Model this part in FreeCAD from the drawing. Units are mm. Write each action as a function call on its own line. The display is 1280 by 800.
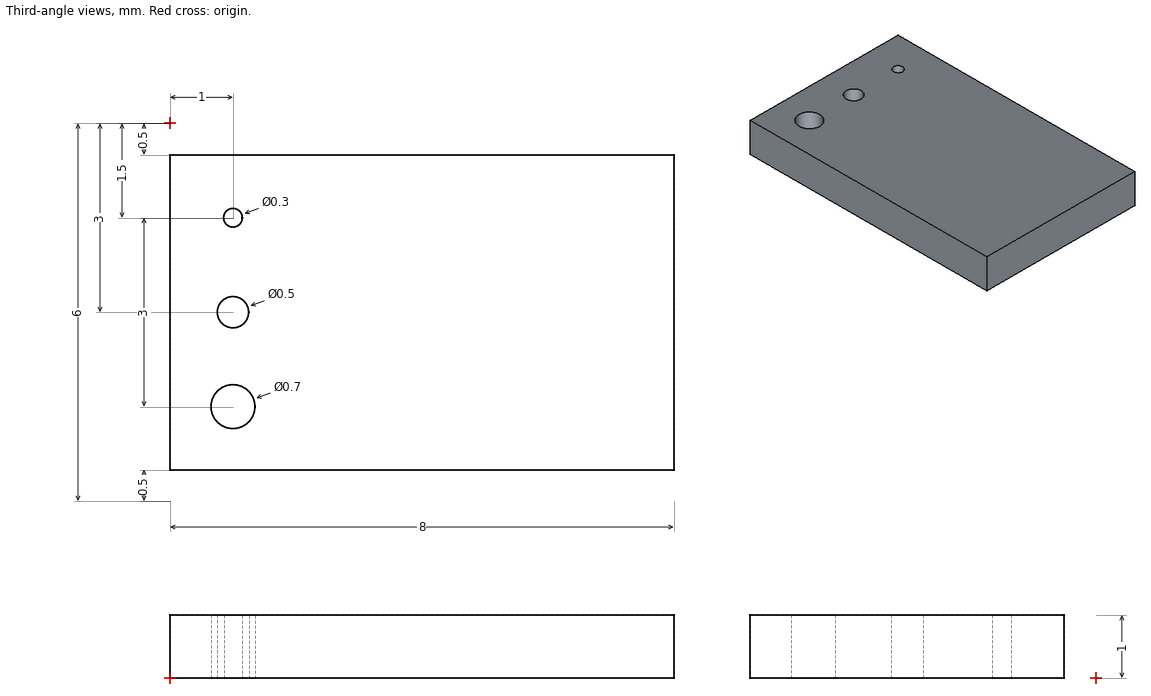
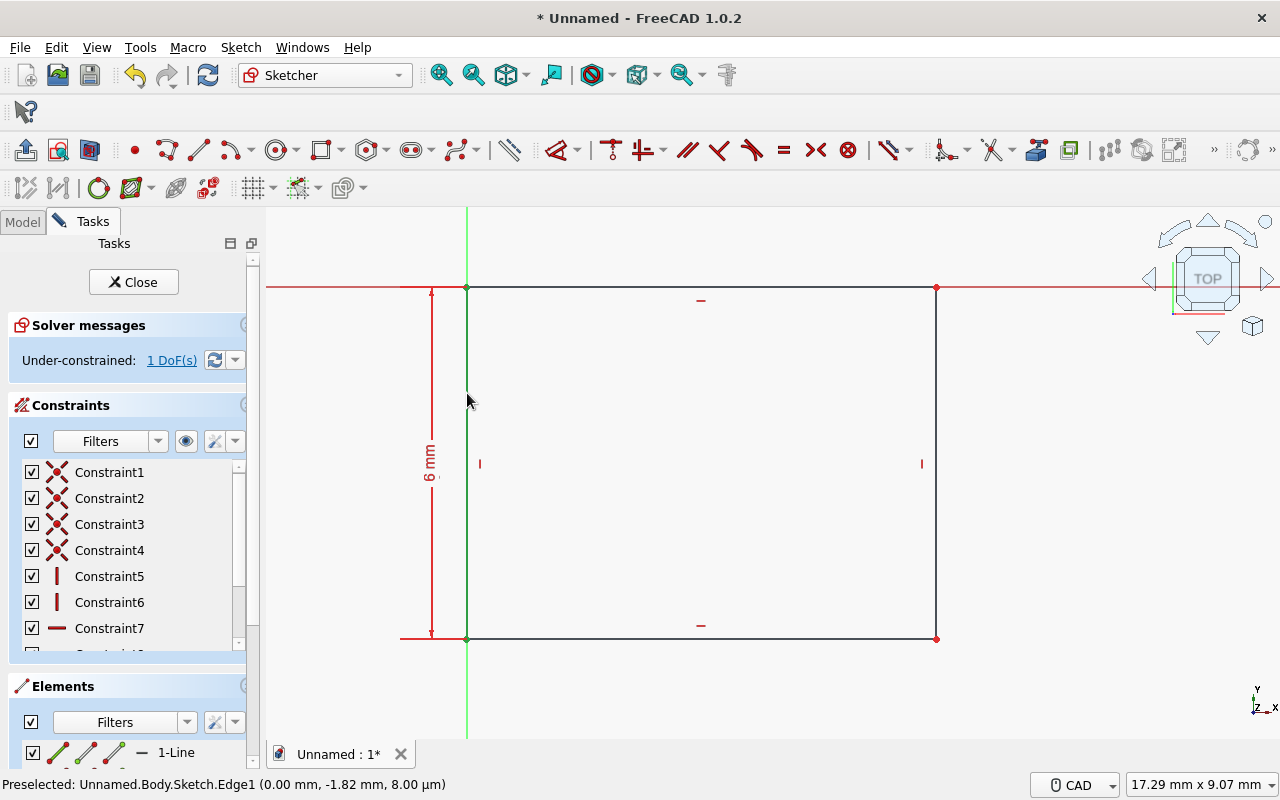
click(608, 639)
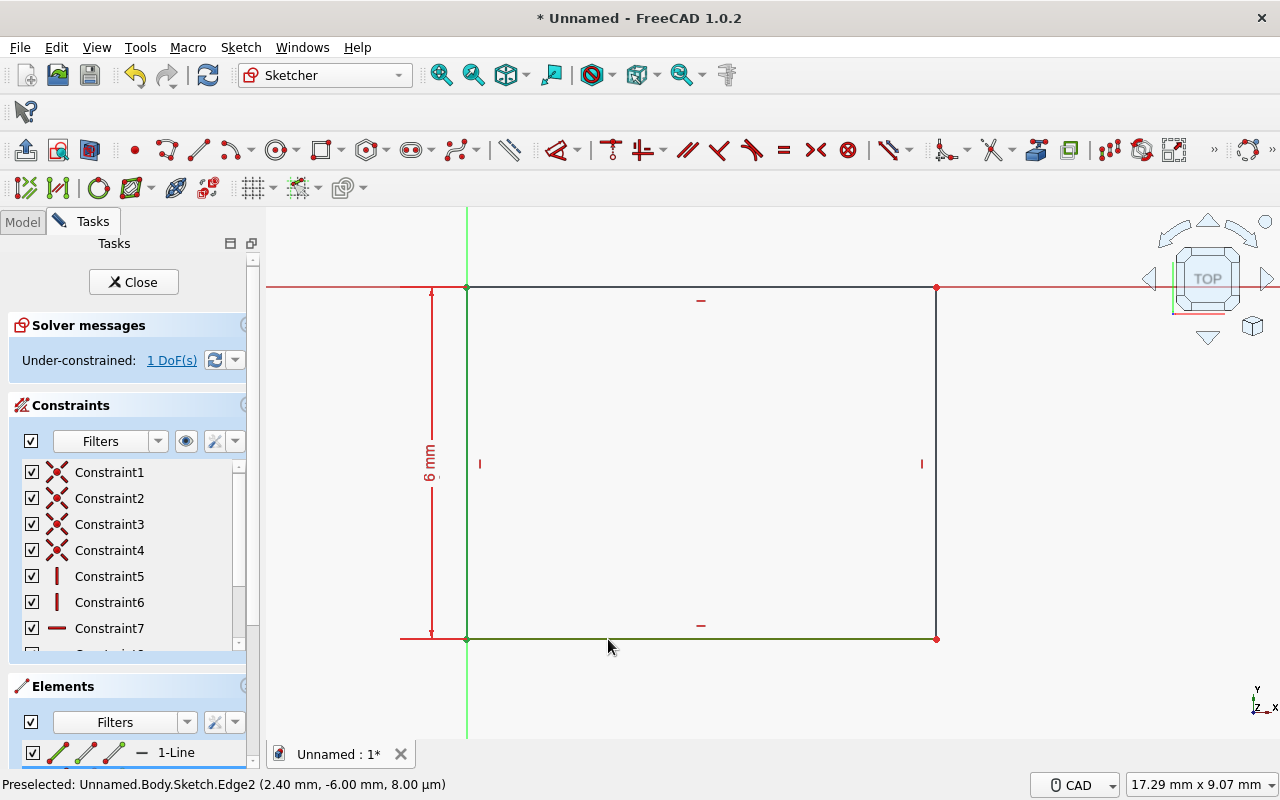
click(580, 150)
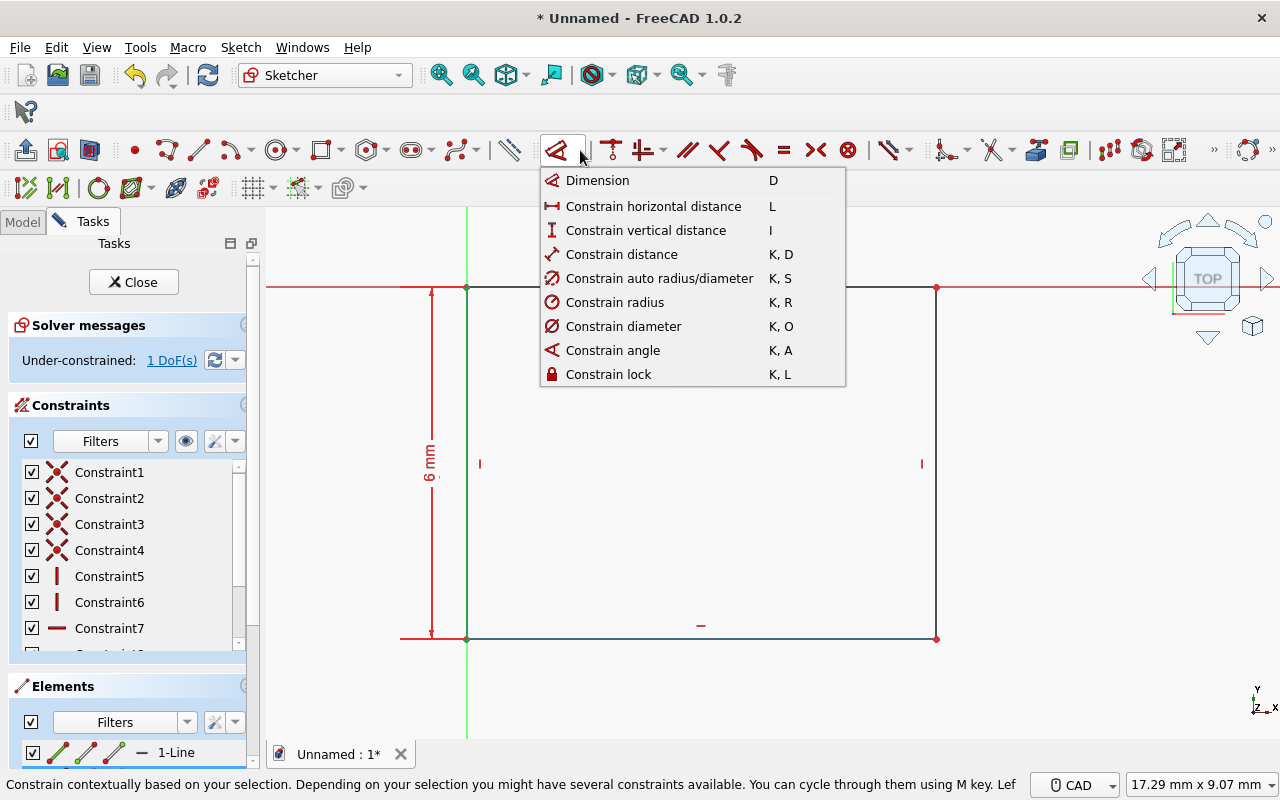
click(693, 206)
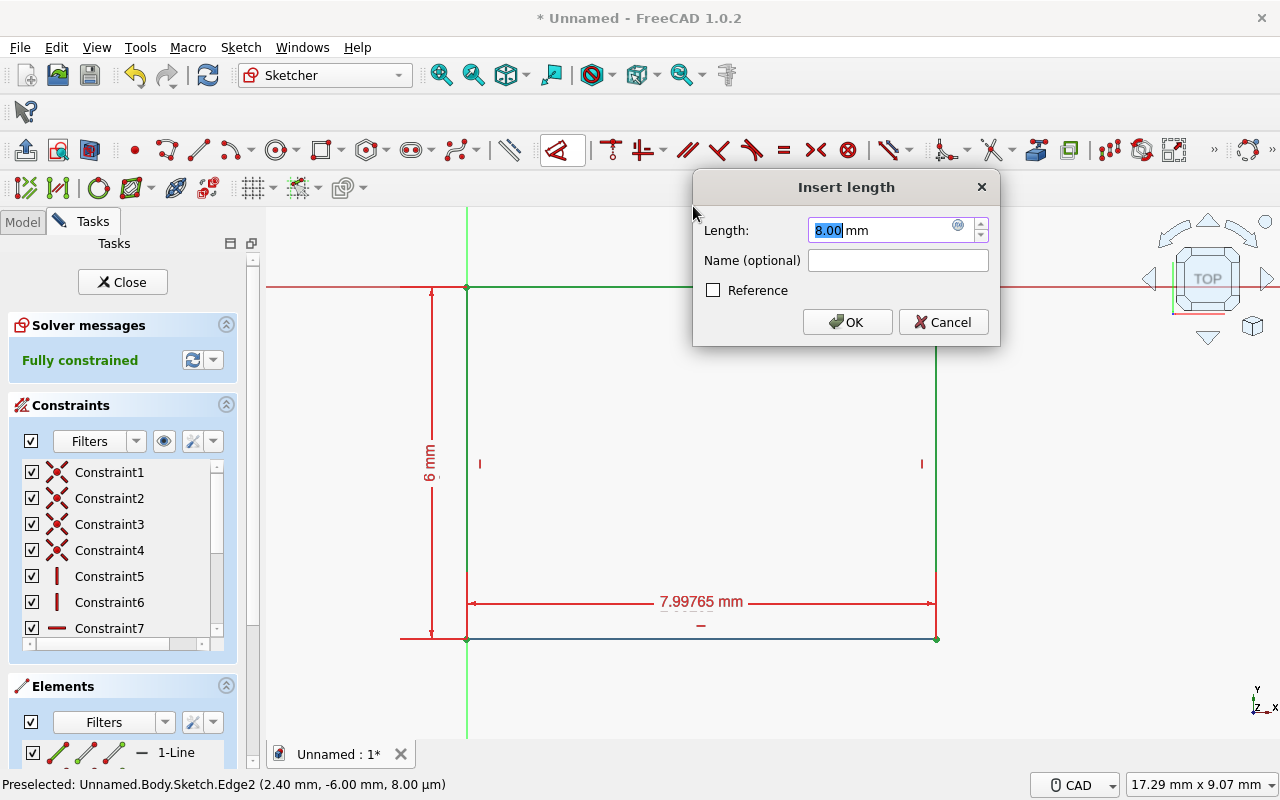
text(8)
key(Return)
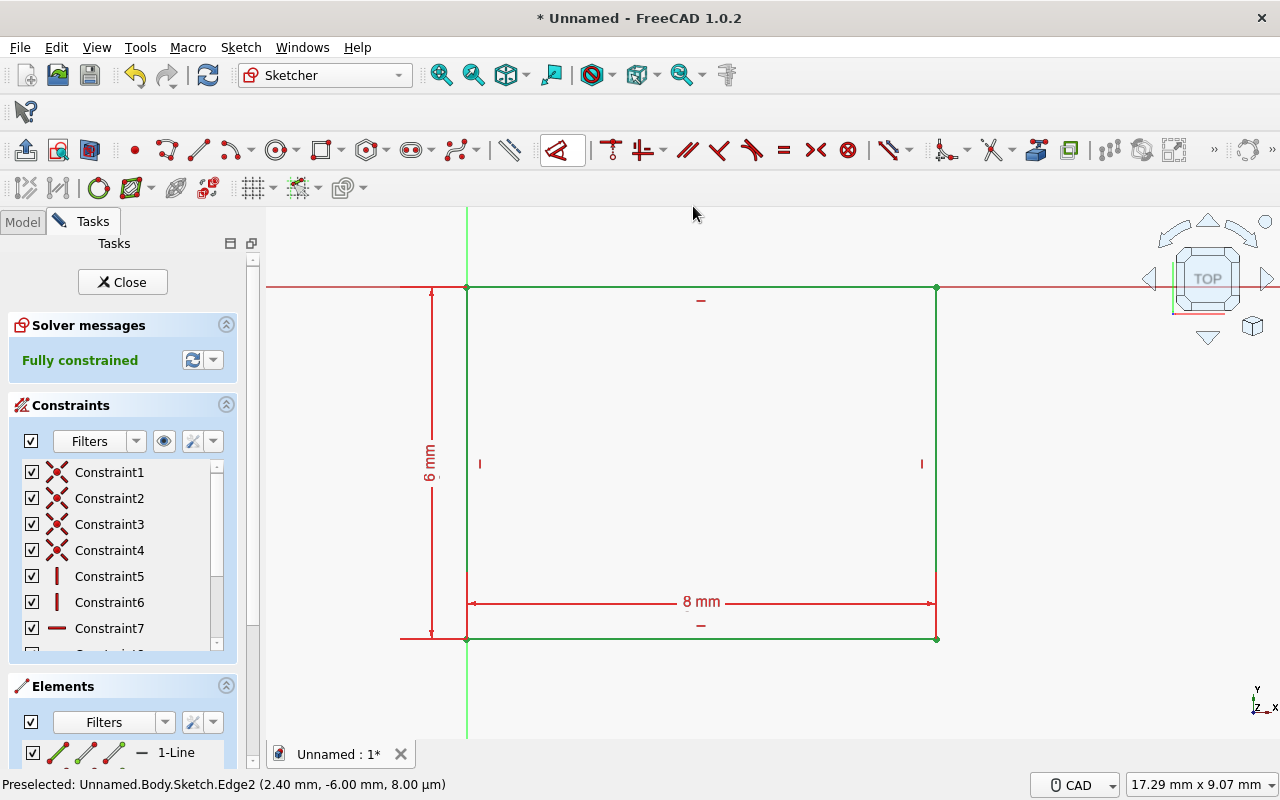
click(123, 282)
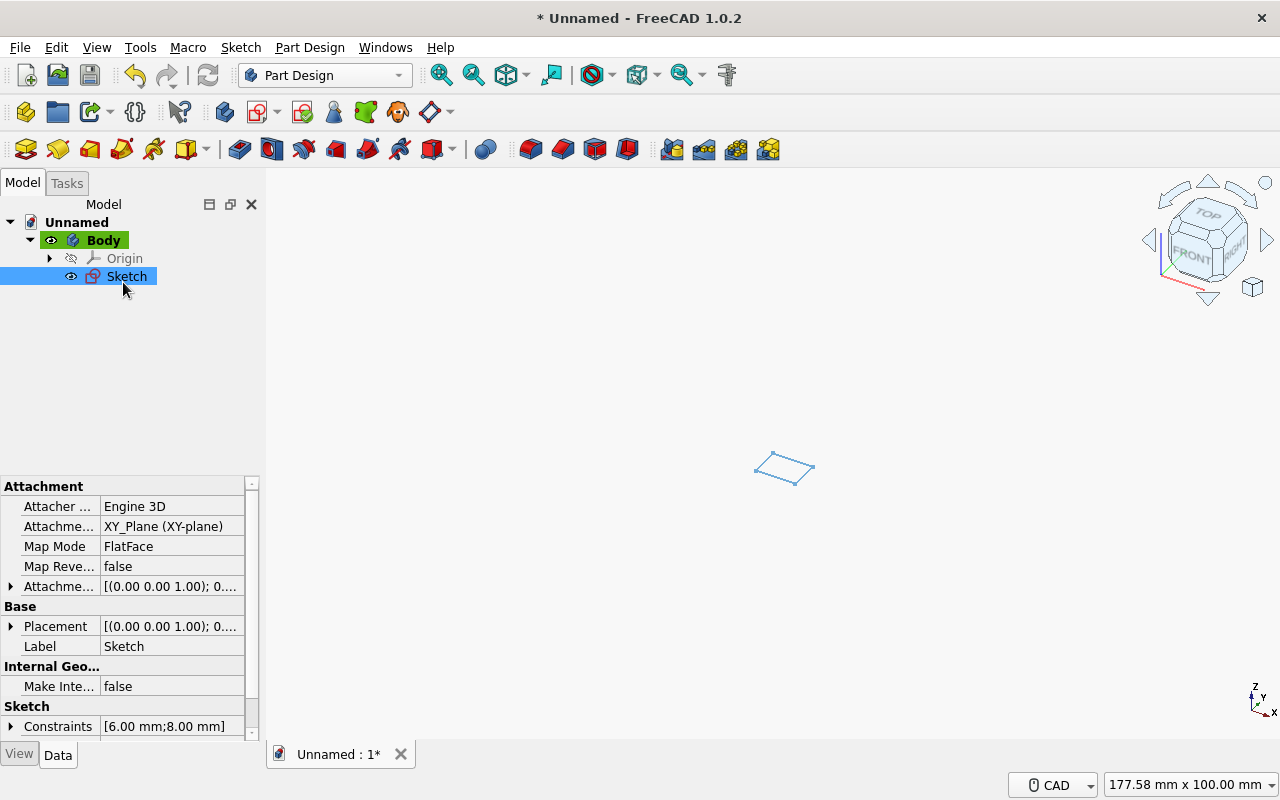
click(26, 150)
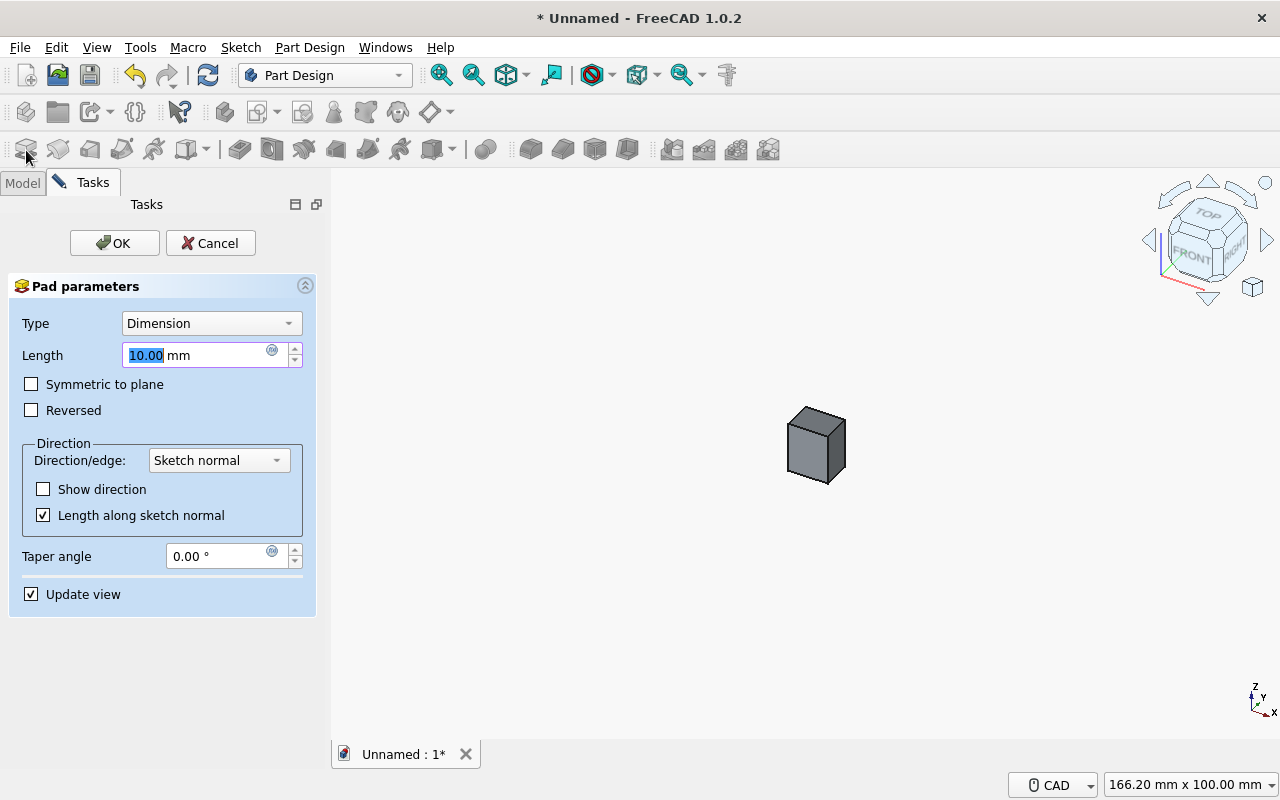
text(1)
key(Tab)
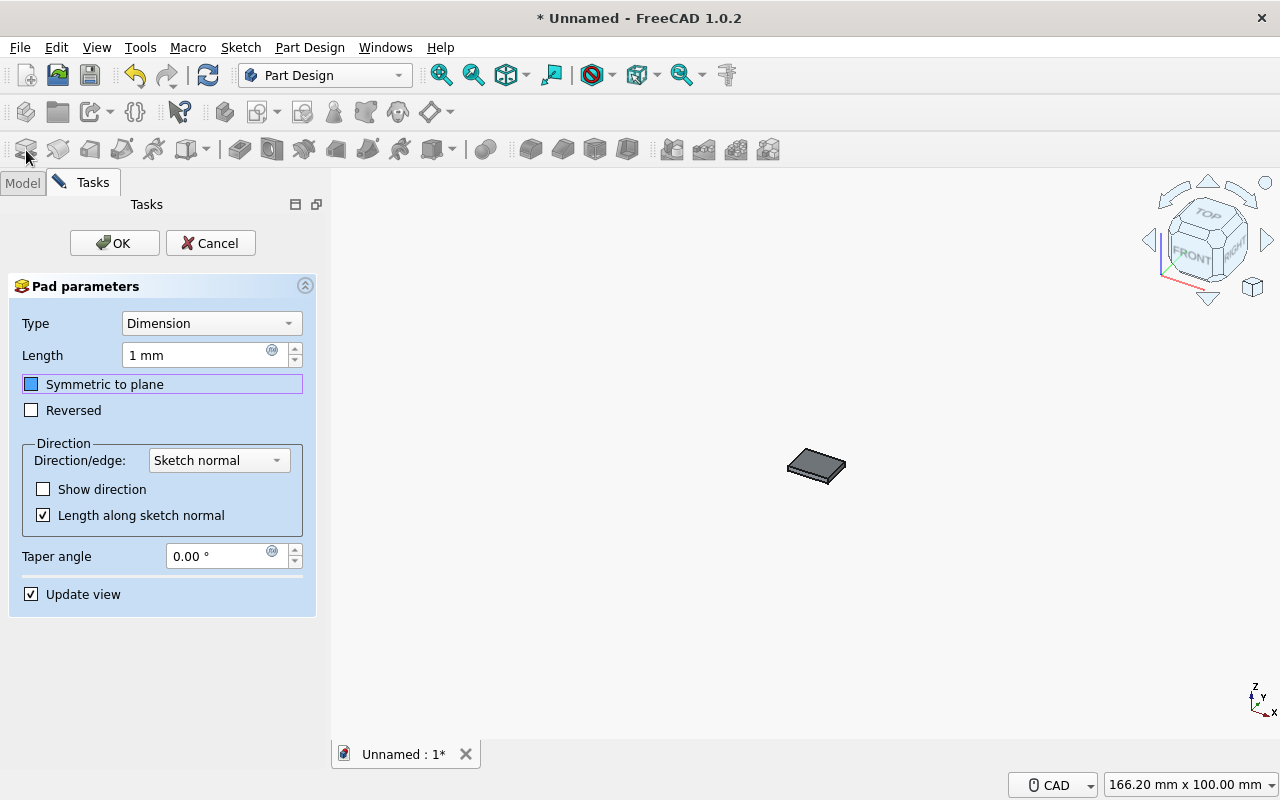
click(115, 243)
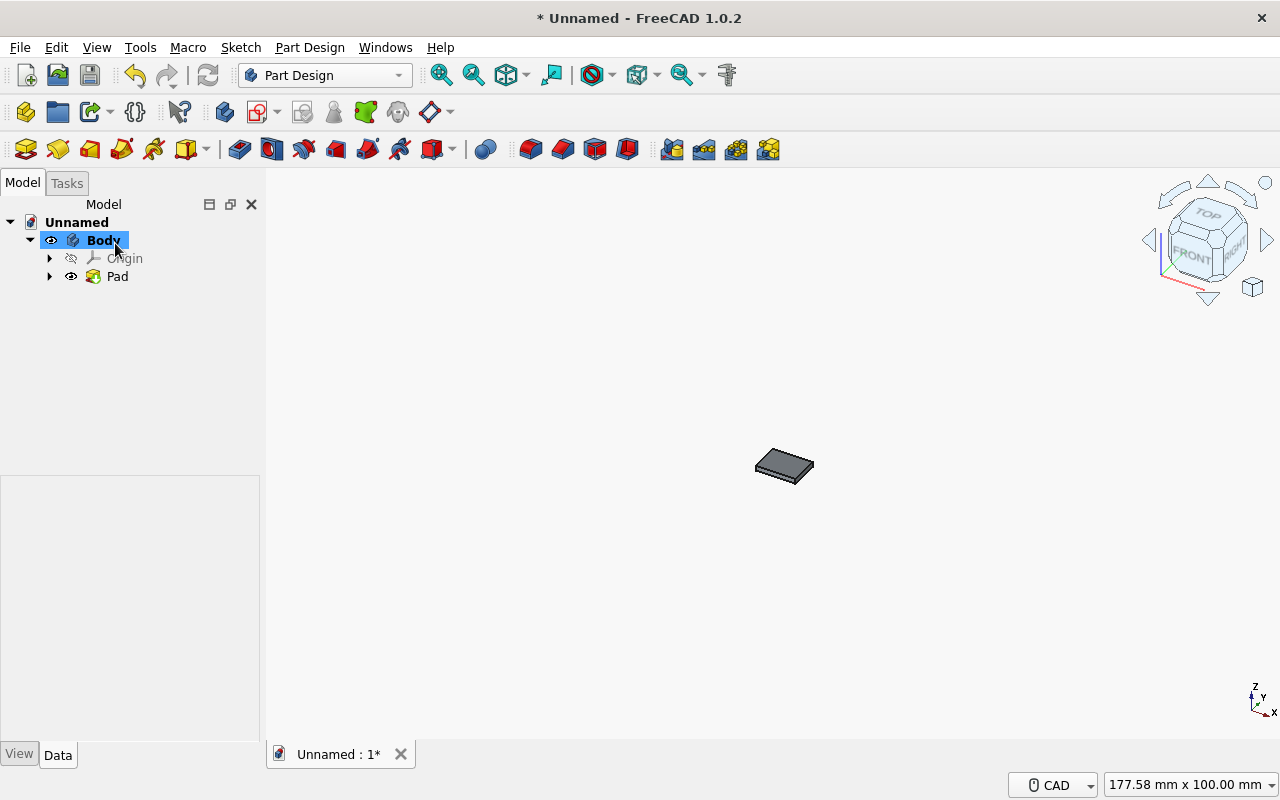
click(442, 76)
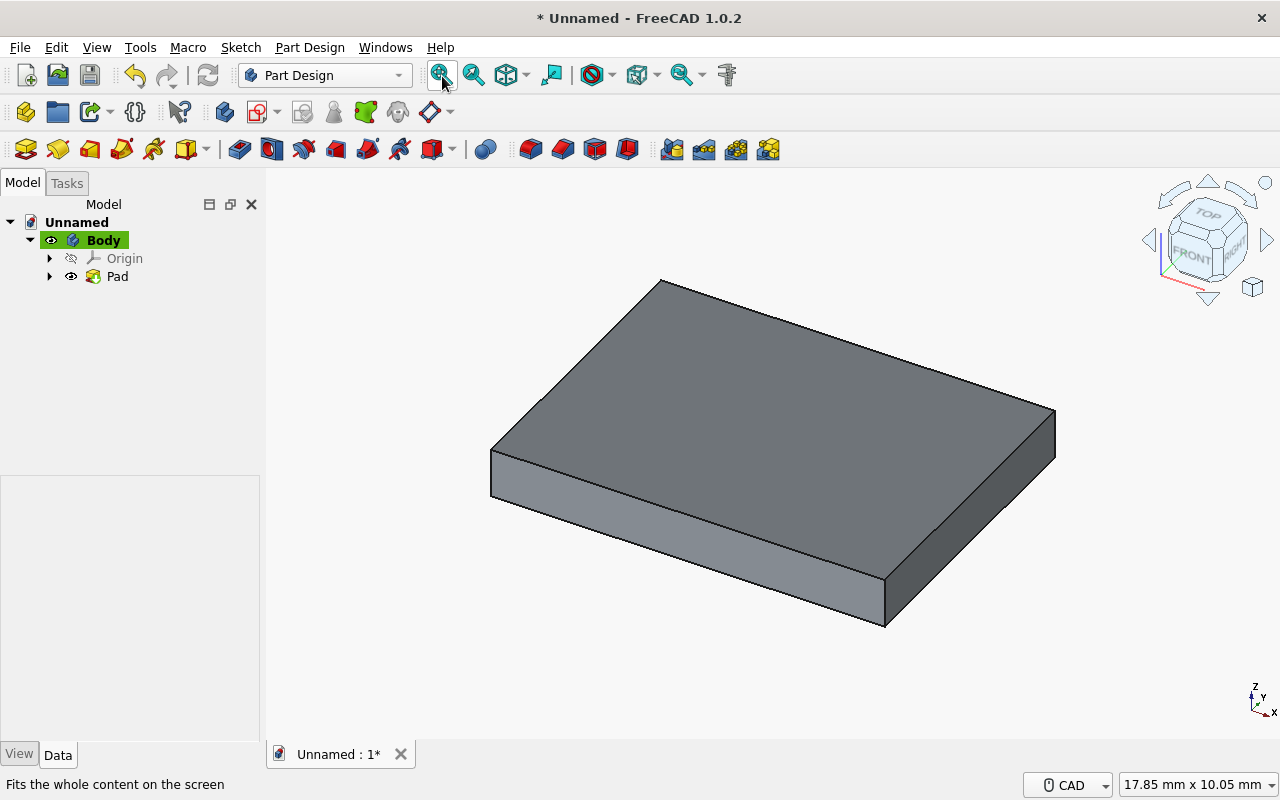
click(773, 429)